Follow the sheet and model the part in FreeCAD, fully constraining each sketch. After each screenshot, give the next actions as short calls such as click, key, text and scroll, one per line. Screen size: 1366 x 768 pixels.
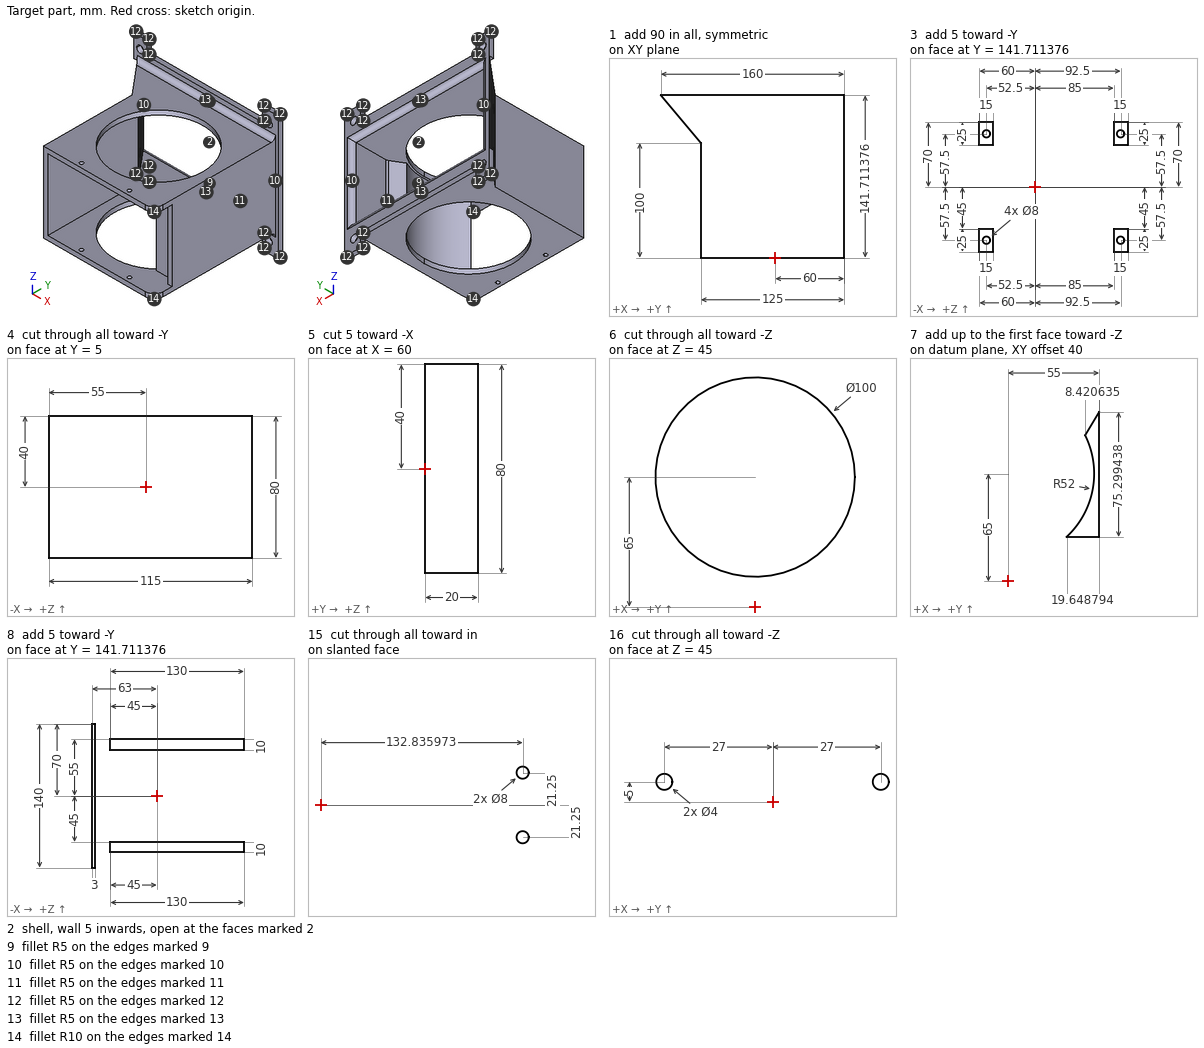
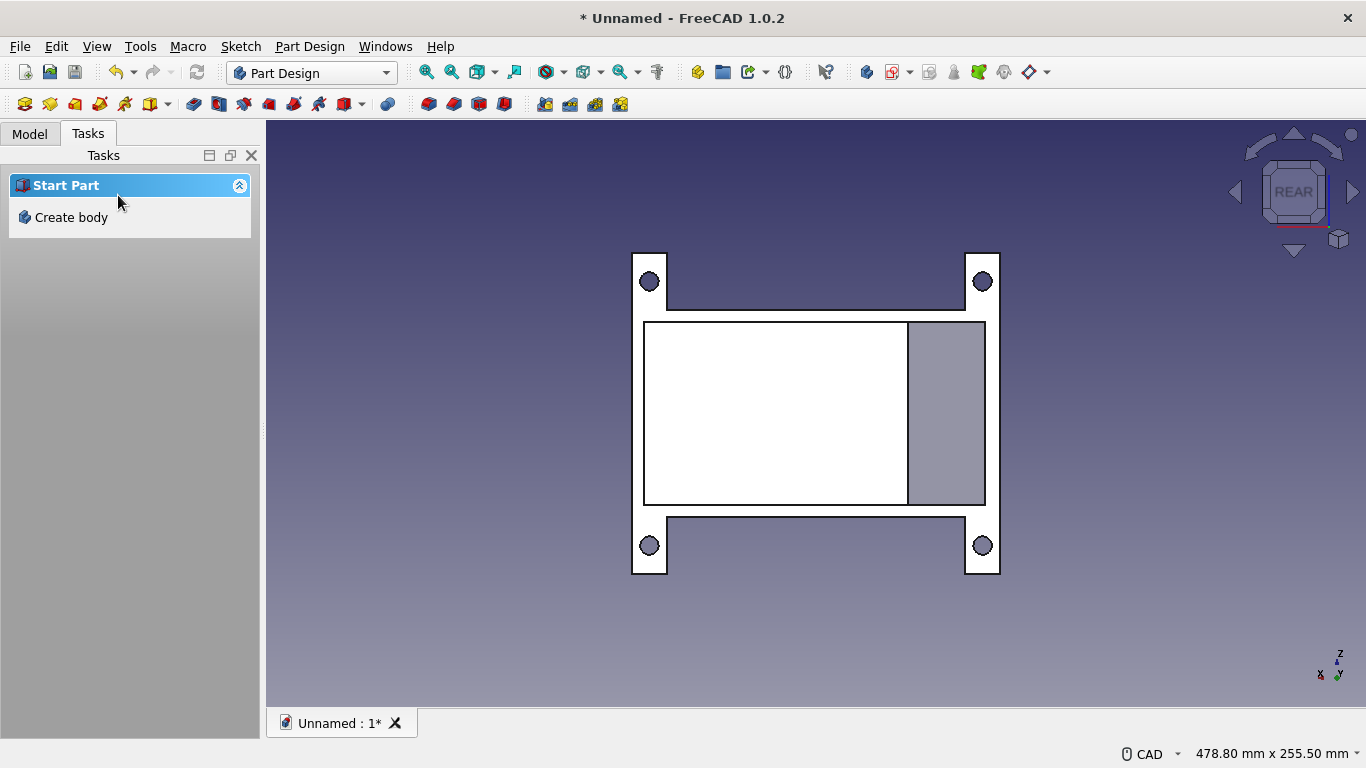
click(738, 412)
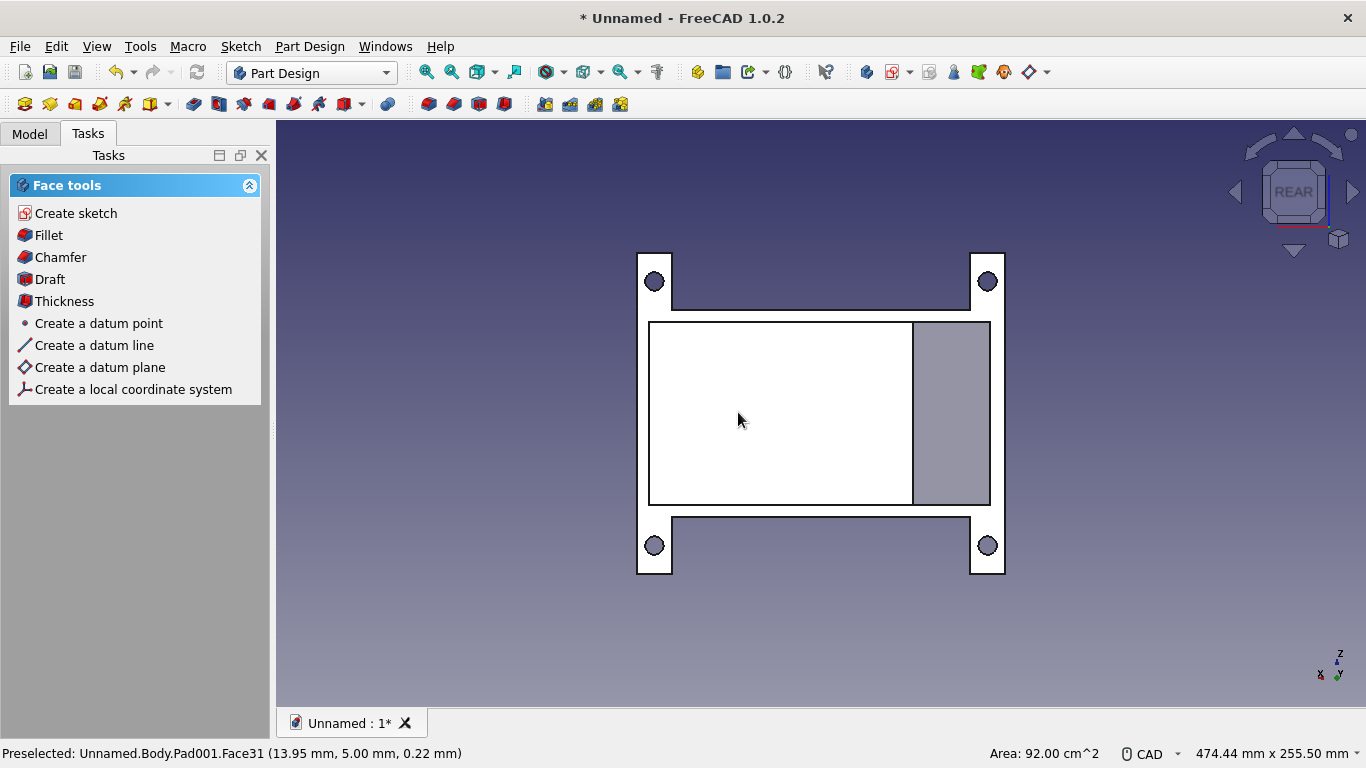
click(892, 72)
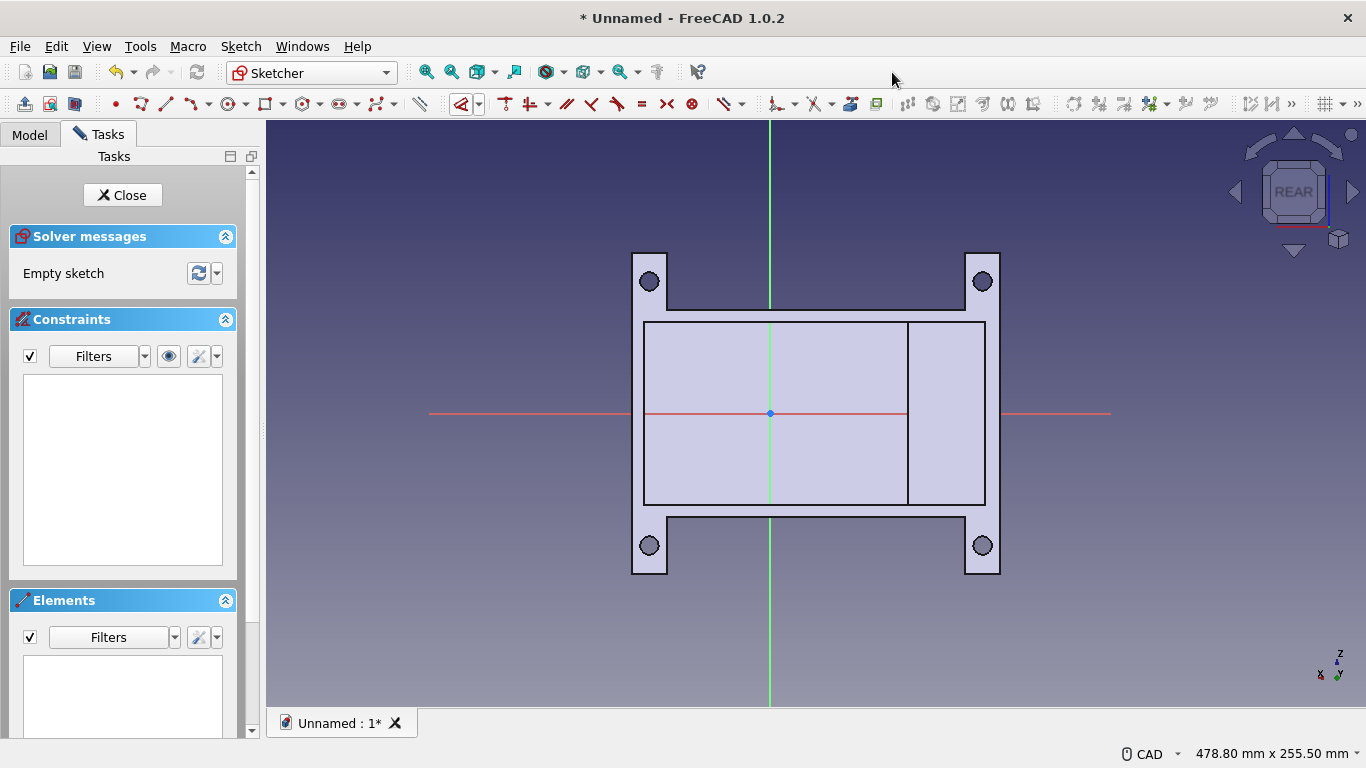
key(q)
key(s)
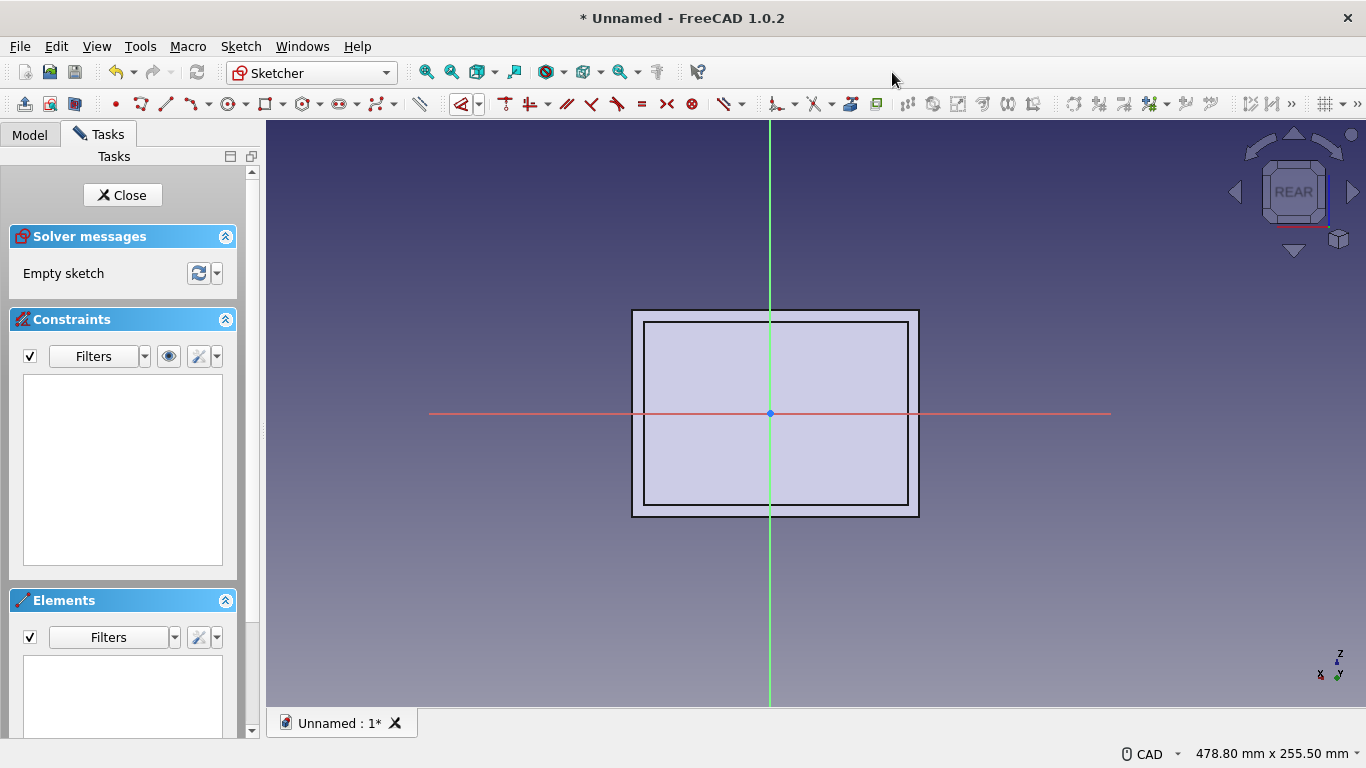
scroll(799, 413, up, 4)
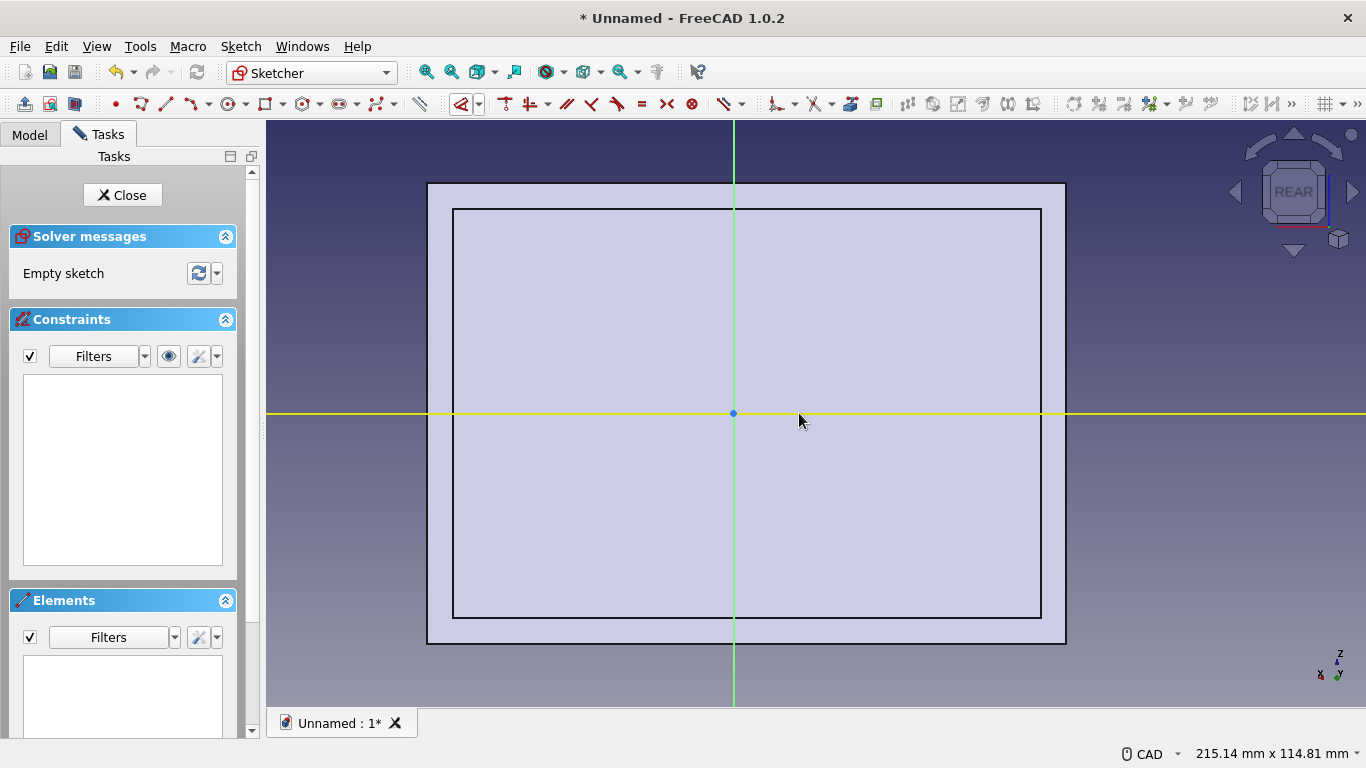
click(264, 104)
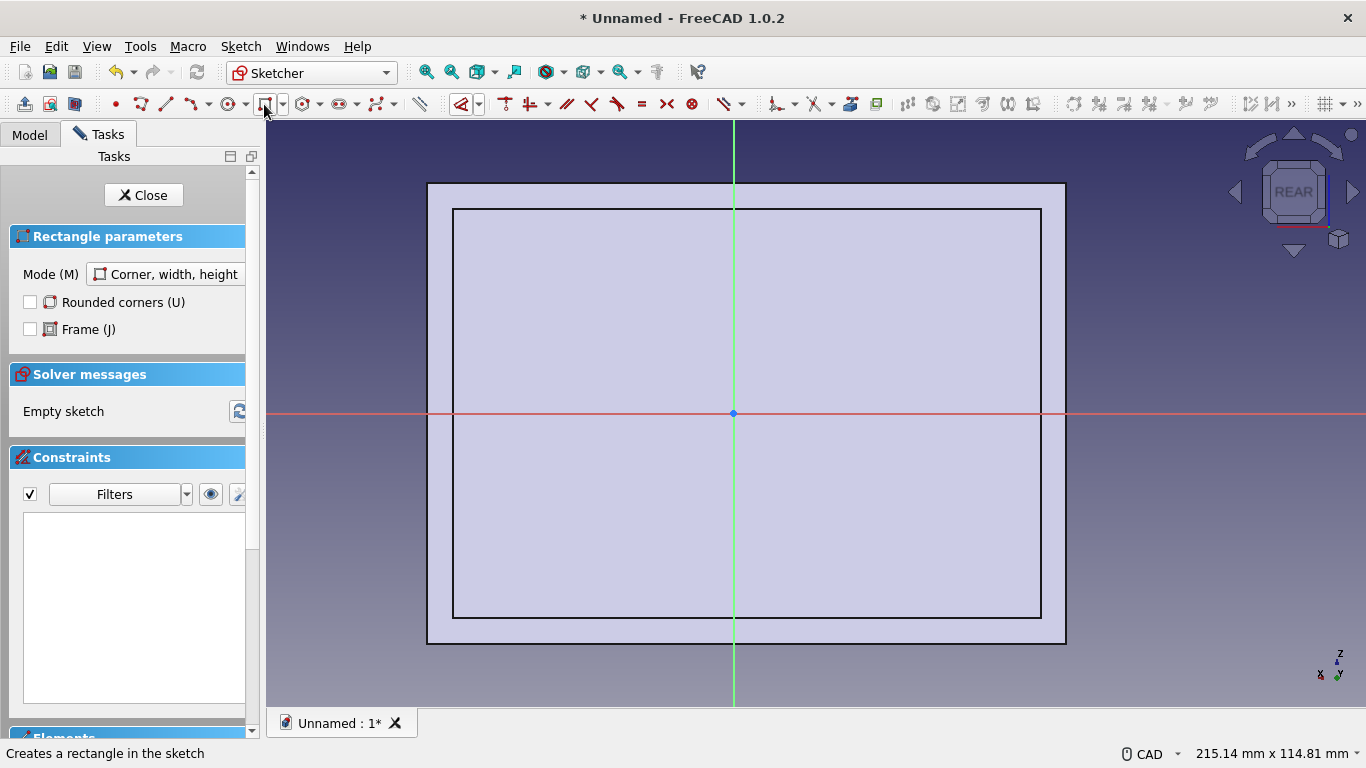
click(453, 209)
move(1041, 618)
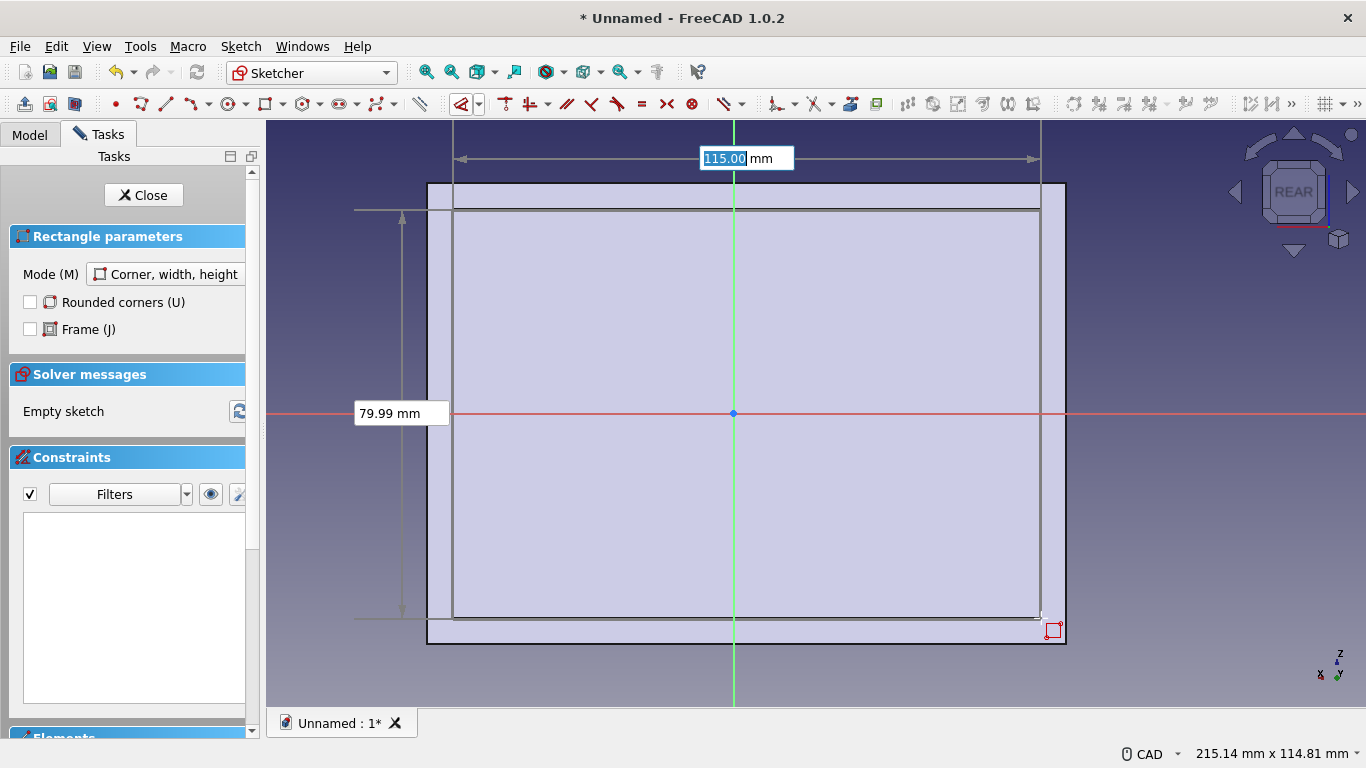
text(115)
key(Tab)
text(80)
key(Return)
key(Escape)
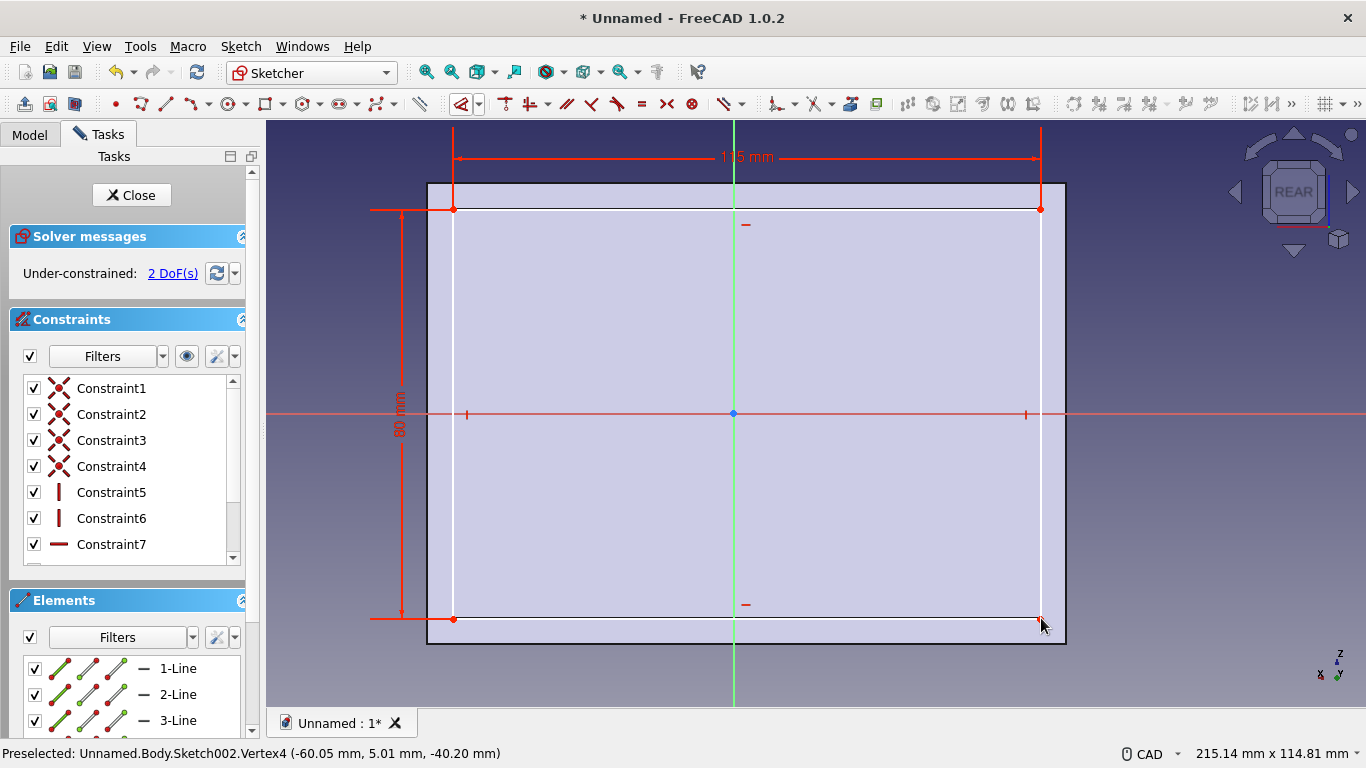
click(453, 210)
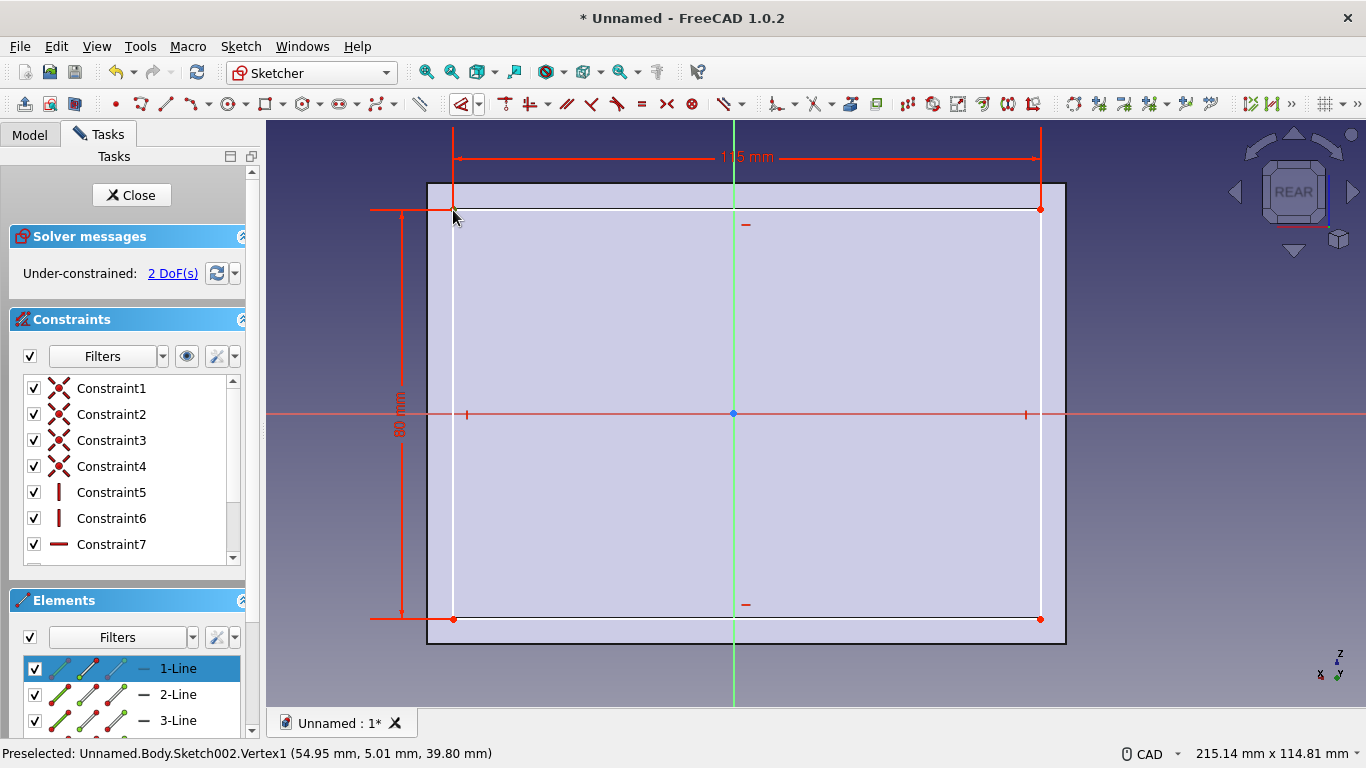
click(478, 104)